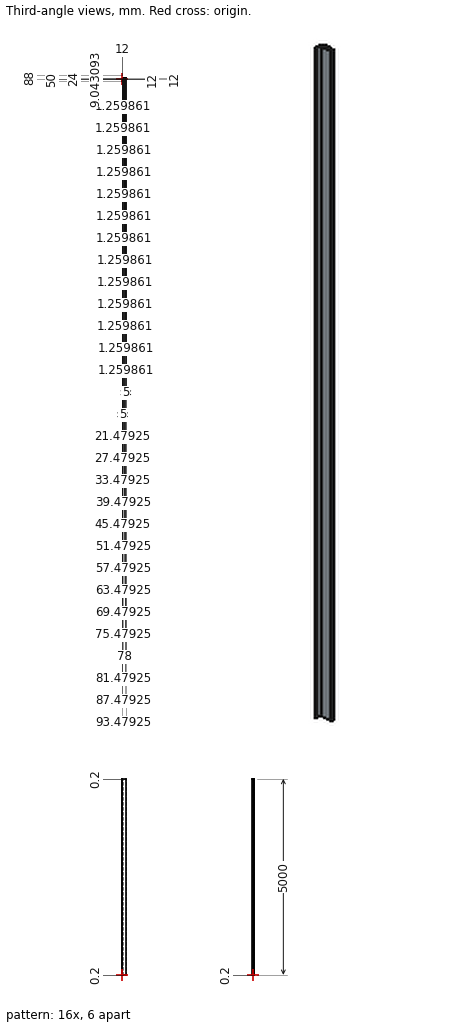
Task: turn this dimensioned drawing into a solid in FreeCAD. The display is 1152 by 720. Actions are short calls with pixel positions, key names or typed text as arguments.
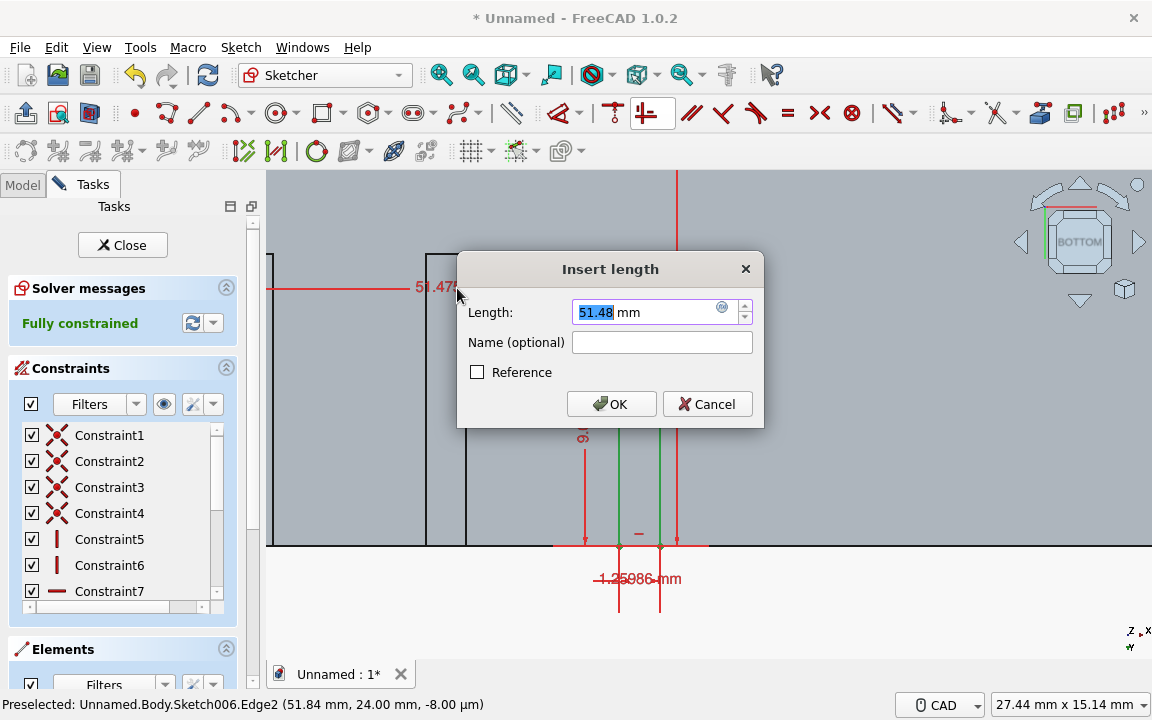
text(51.47925)
key(Return)
key(Escape)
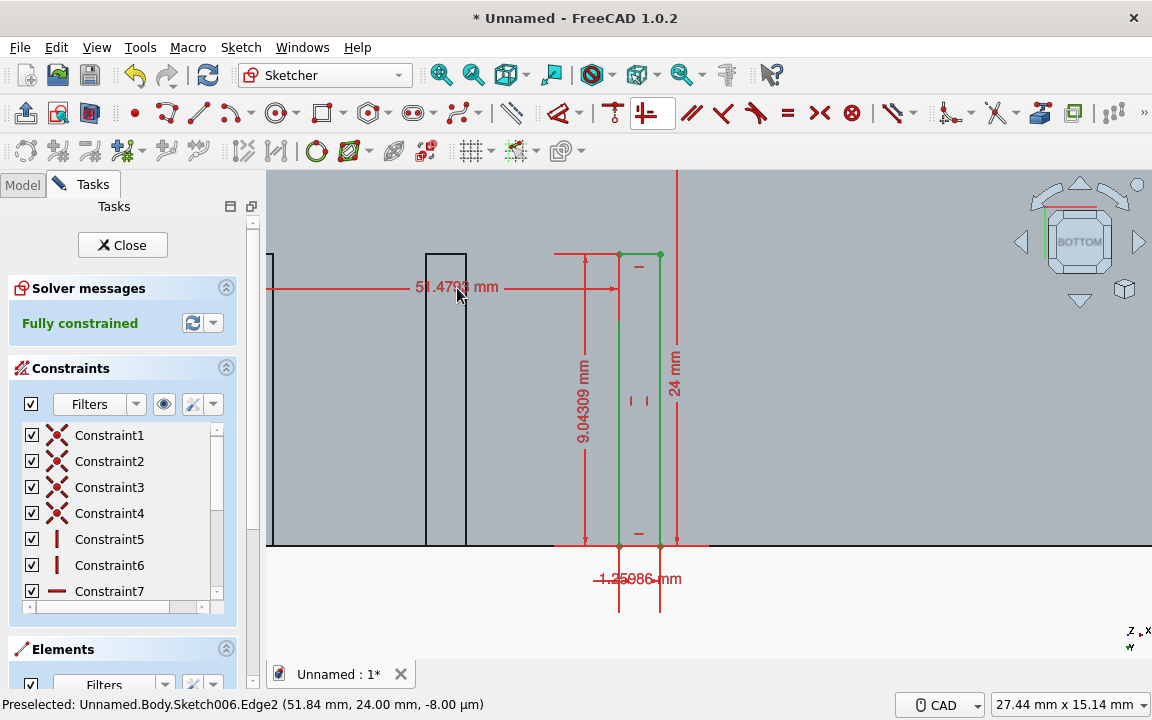
click(123, 245)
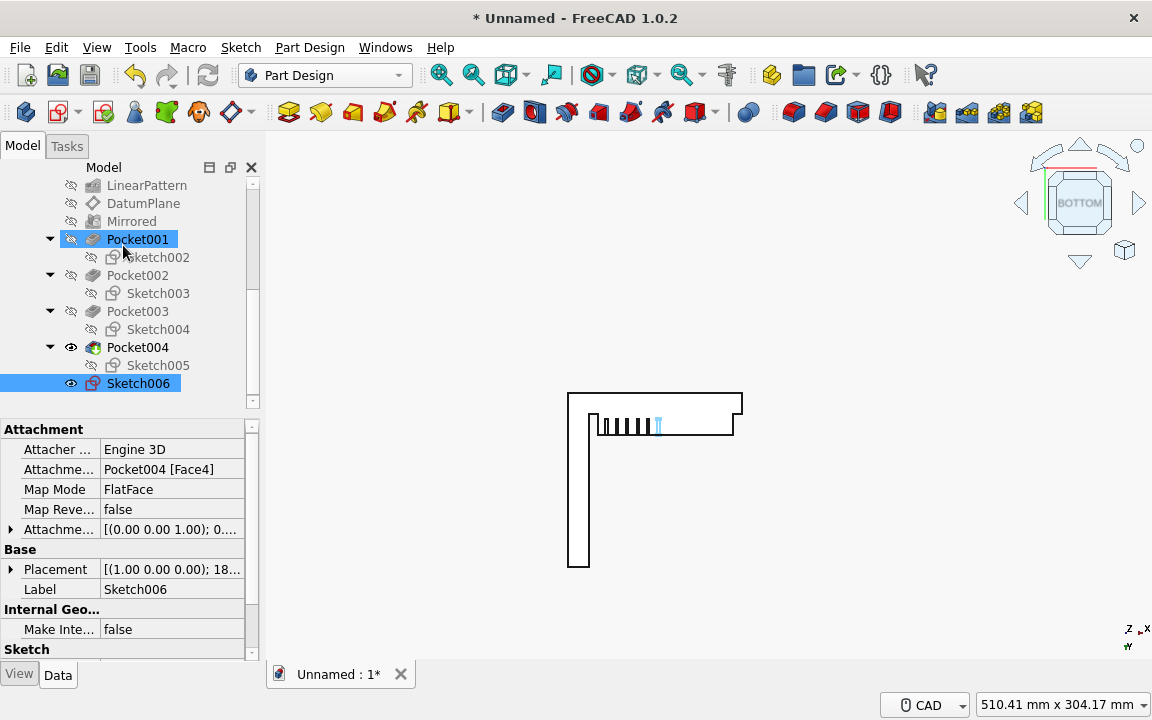
click(504, 112)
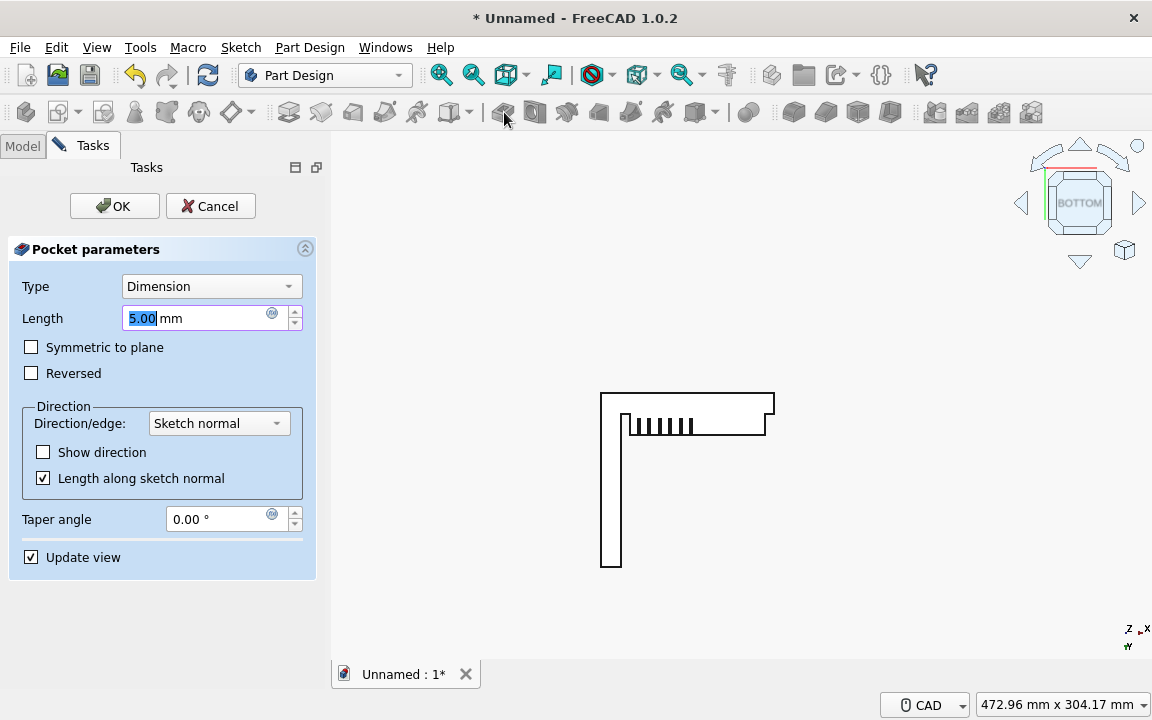
text(0.2)
key(Tab)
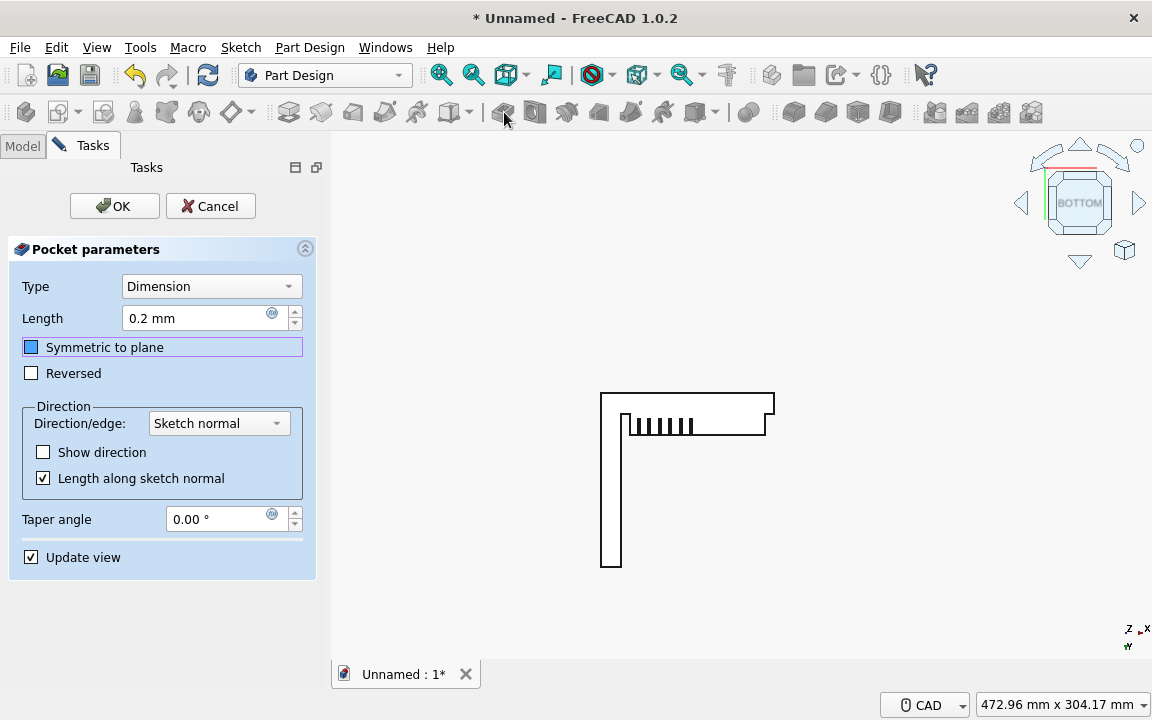
click(115, 206)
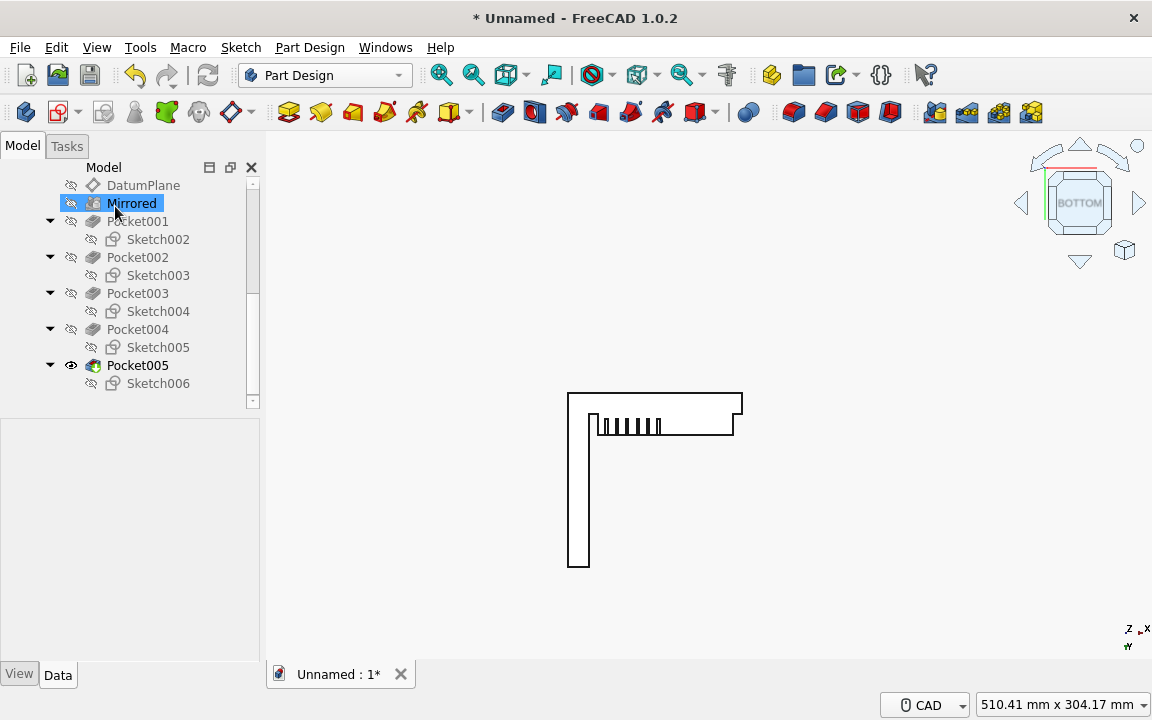
click(442, 76)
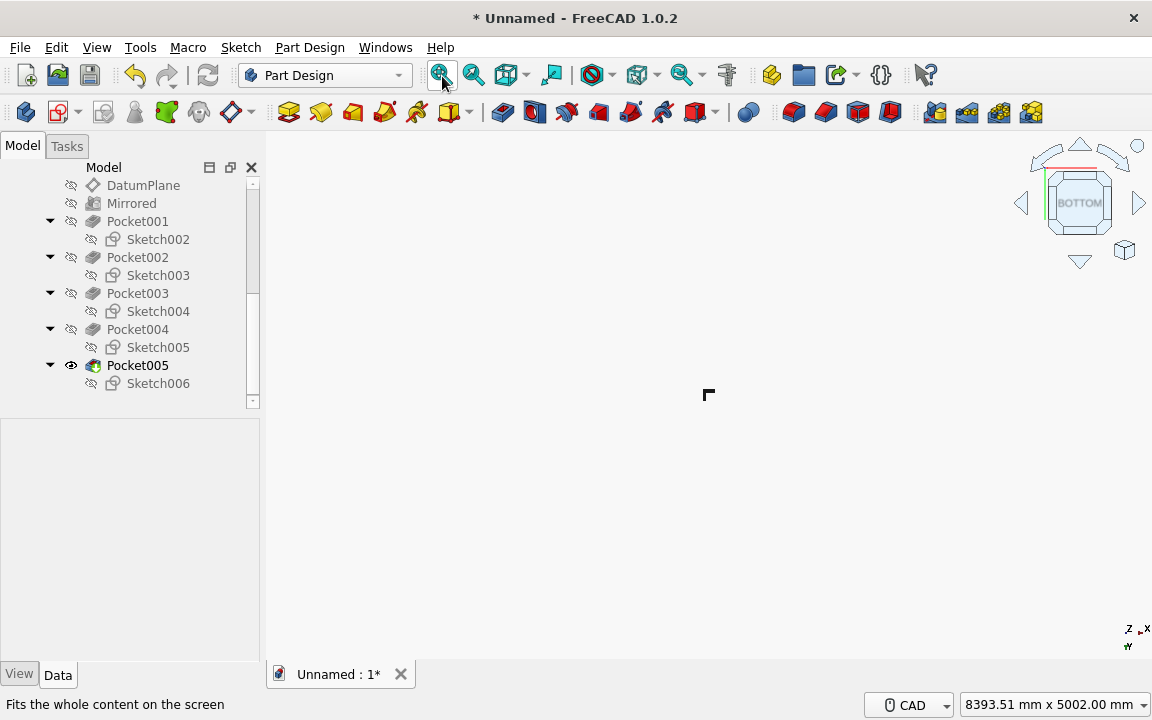
click(58, 112)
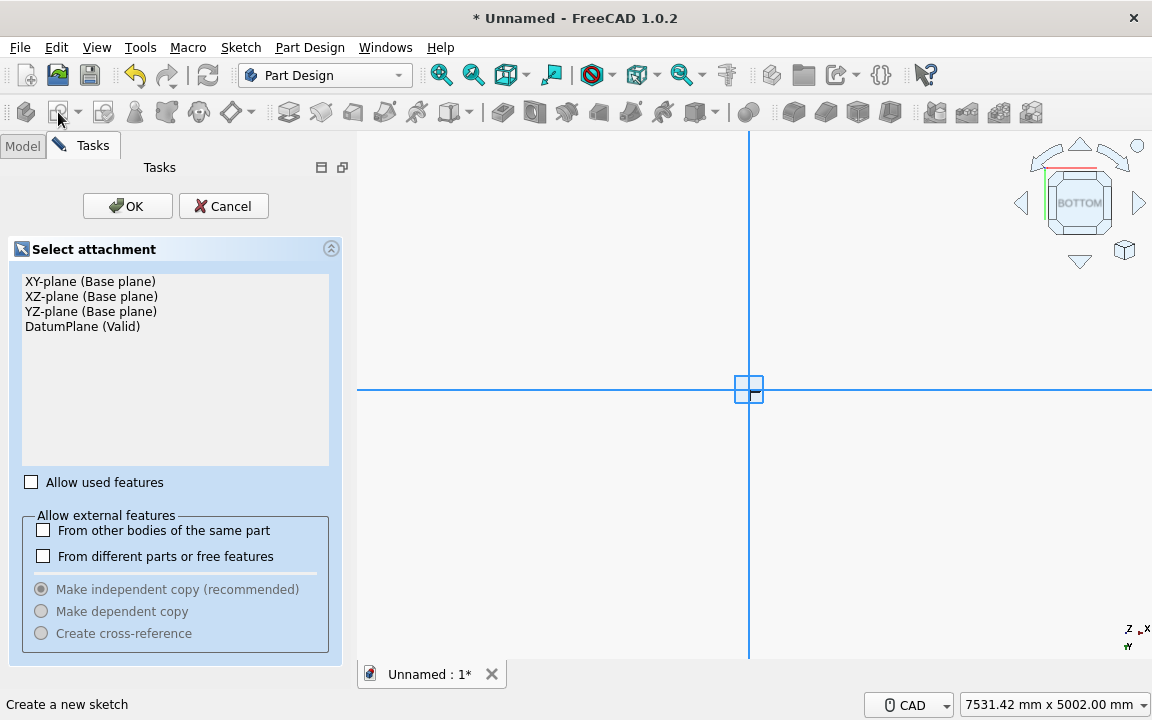
click(82, 282)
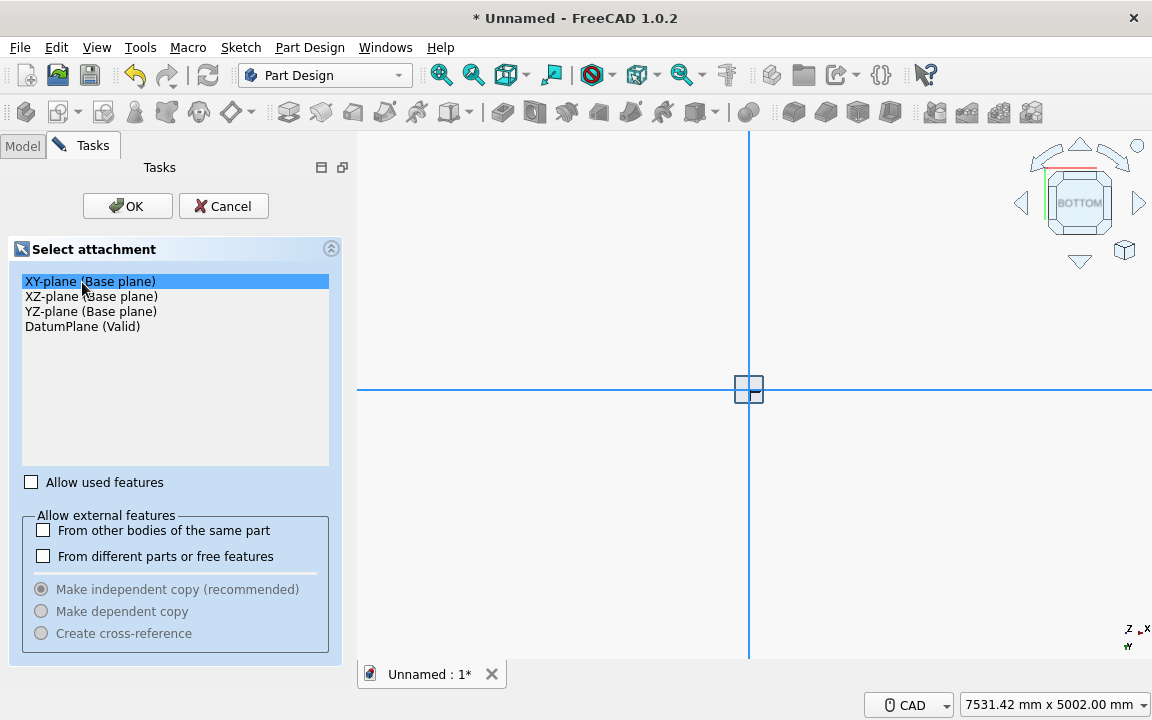
click(128, 206)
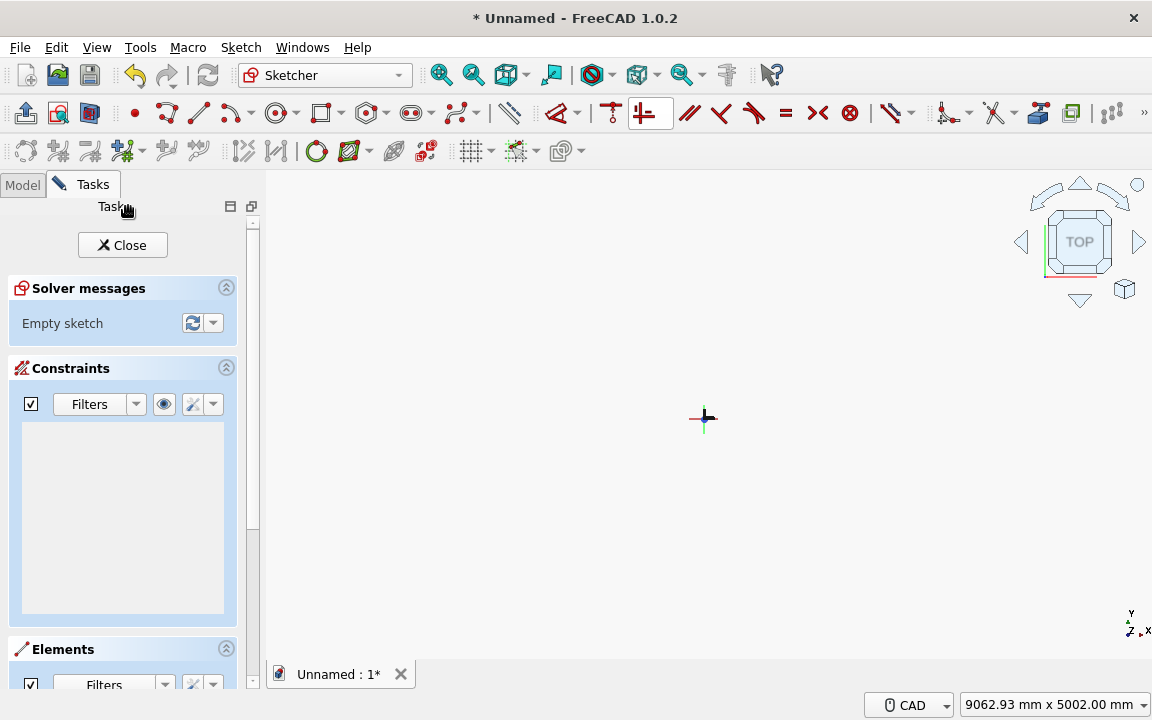
click(90, 114)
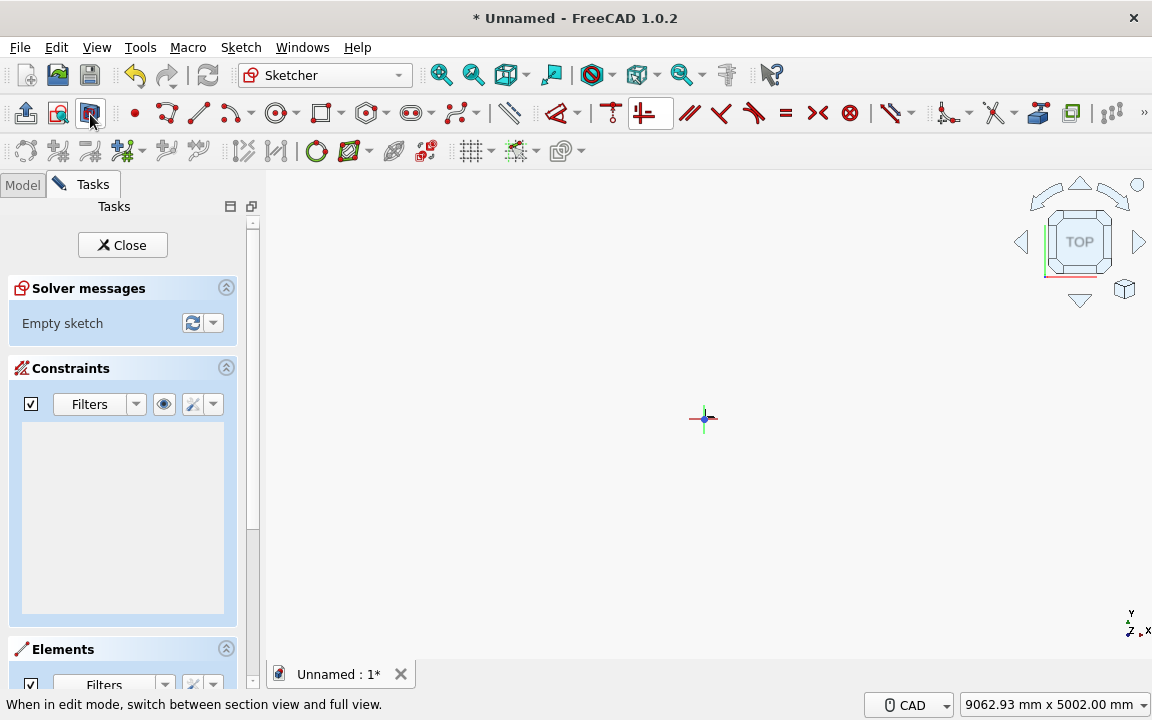
scroll(713, 418, up, 15)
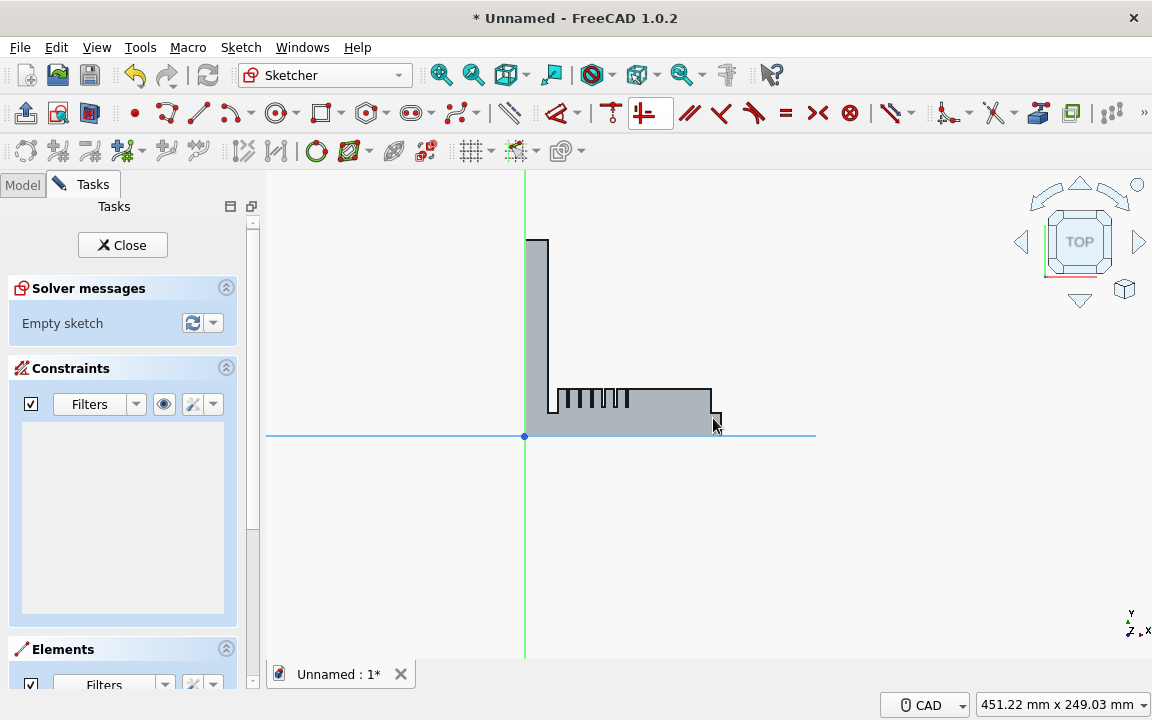
scroll(639, 397, up, 14)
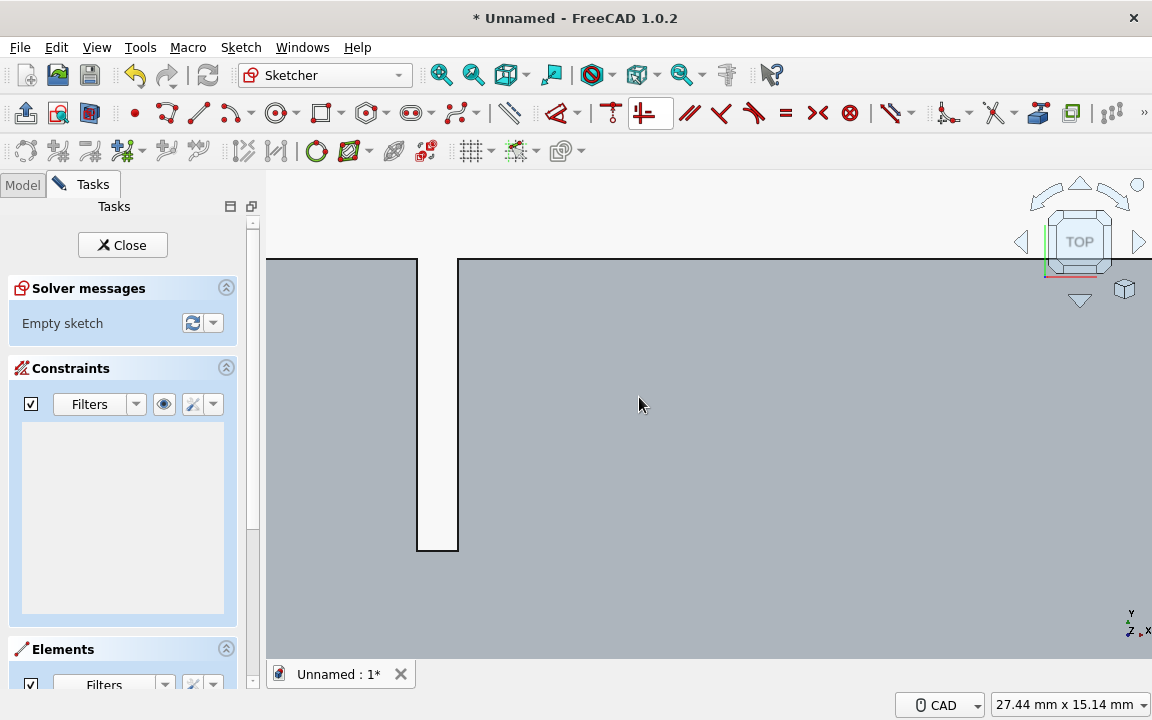
click(322, 114)